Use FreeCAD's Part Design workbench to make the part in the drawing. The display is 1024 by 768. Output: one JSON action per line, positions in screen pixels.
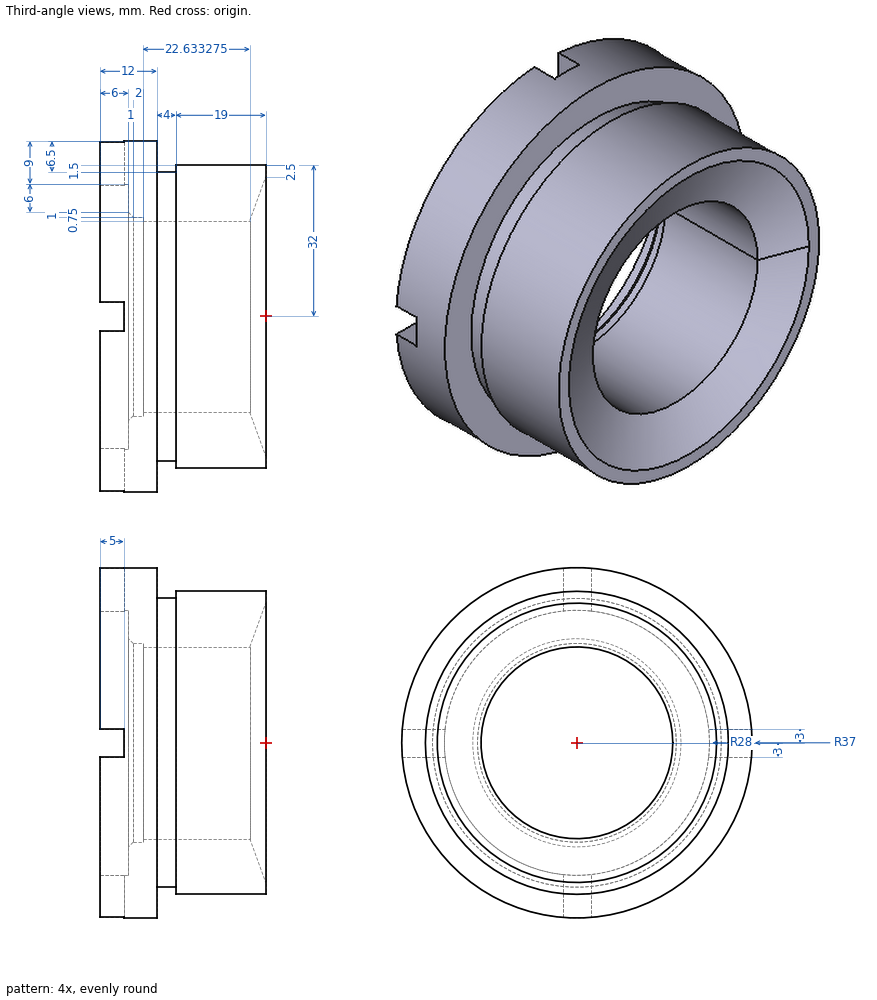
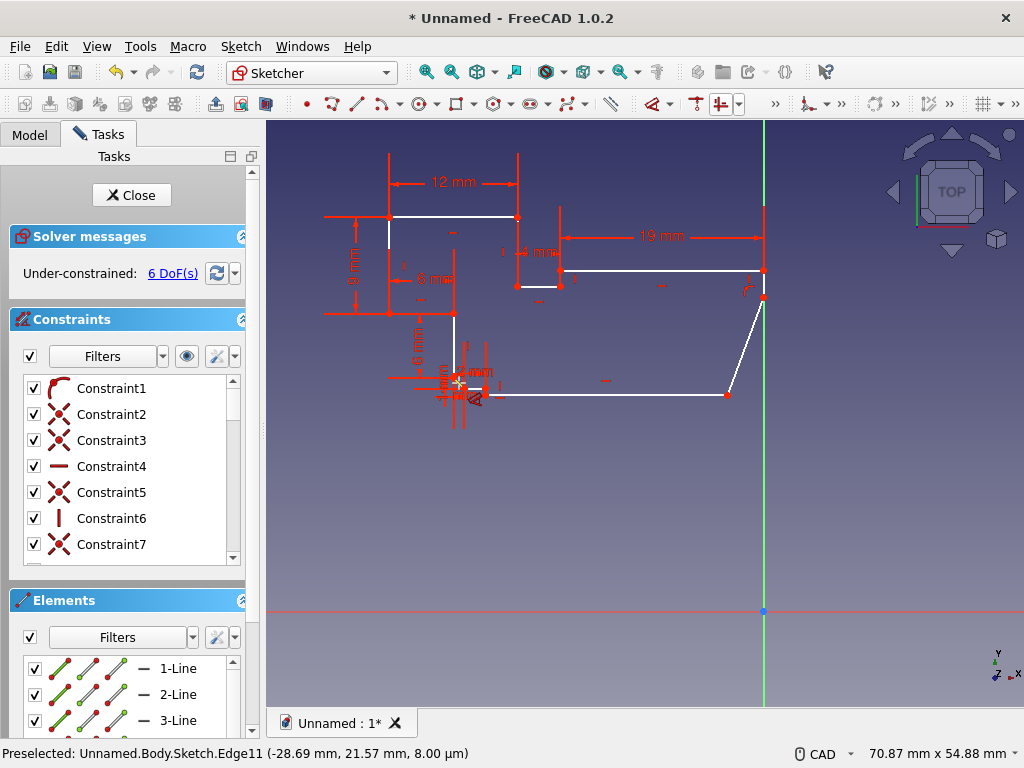
{"action": "scroll", "coordinate": [764, 289], "scroll_direction": "up", "scroll_amount": 3}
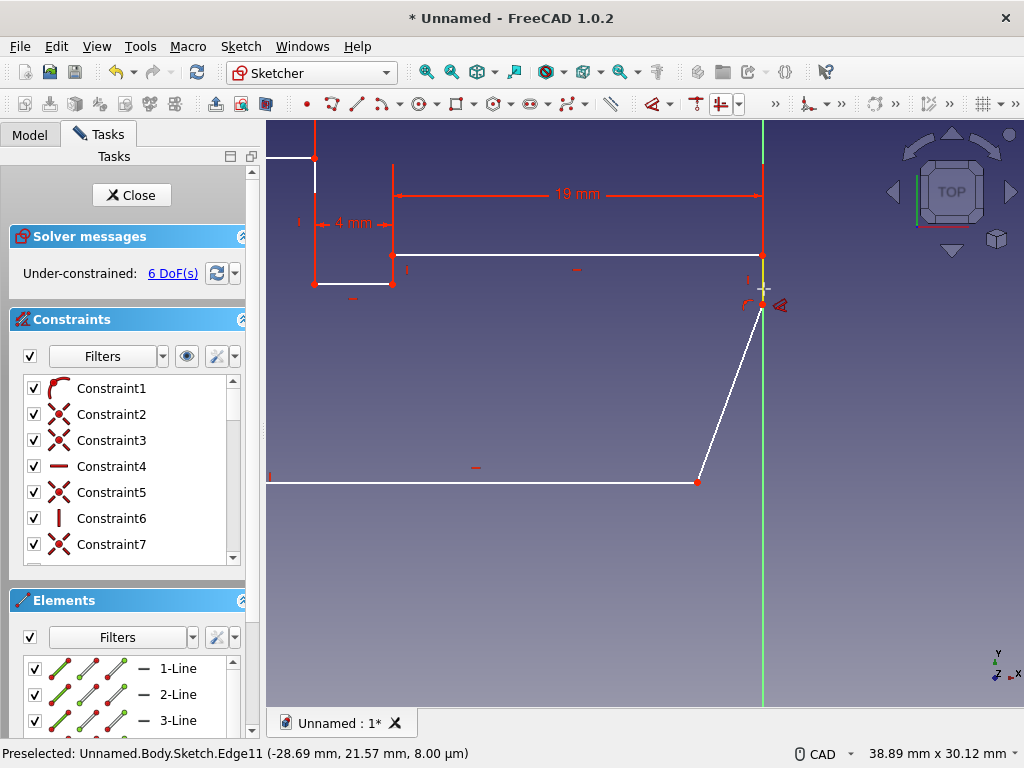
{"action": "left_click", "coordinate": [763, 290]}
{"action": "left_click", "coordinate": [797, 280]}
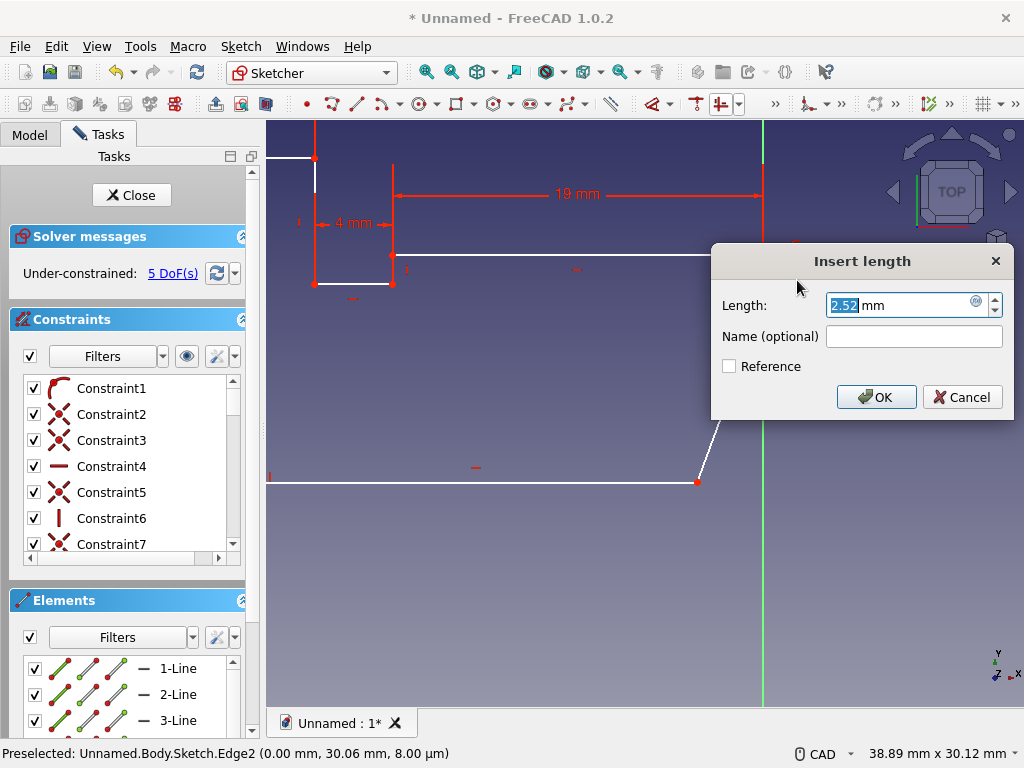
{"action": "type", "text": "2.5"}
{"action": "key", "text": "Return"}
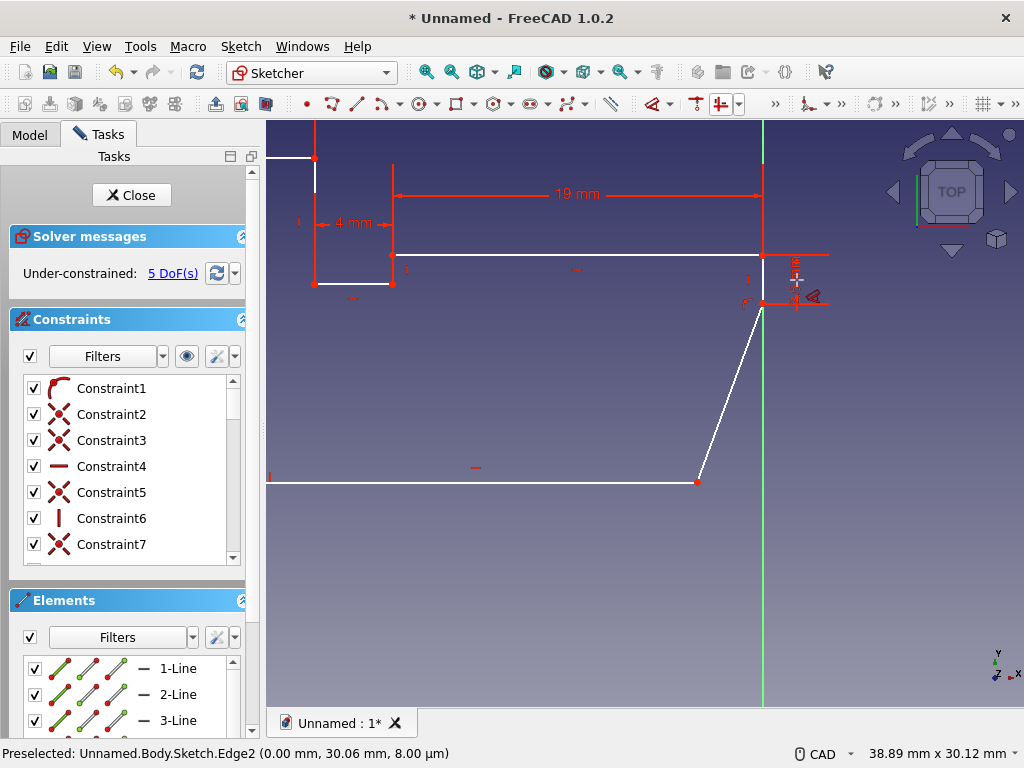
{"action": "scroll", "coordinate": [393, 267], "scroll_direction": "up", "scroll_amount": 2}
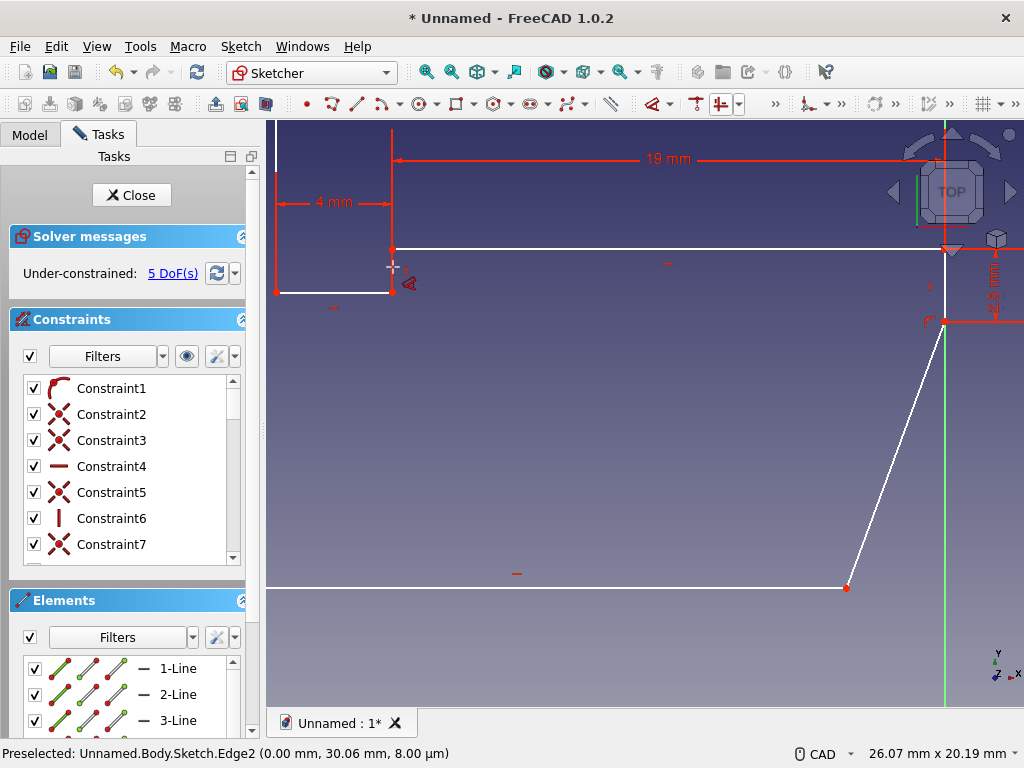
{"action": "left_click", "coordinate": [392, 267]}
{"action": "left_click", "coordinate": [358, 271]}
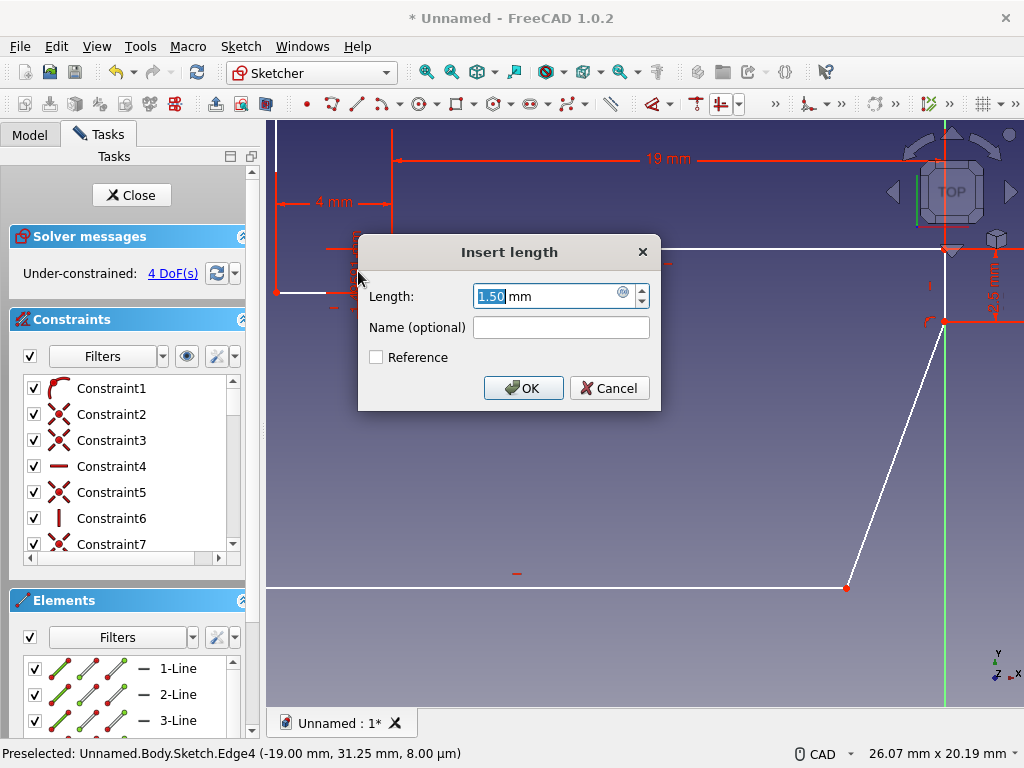
{"action": "type", "text": "1.5"}
{"action": "key", "text": "Return"}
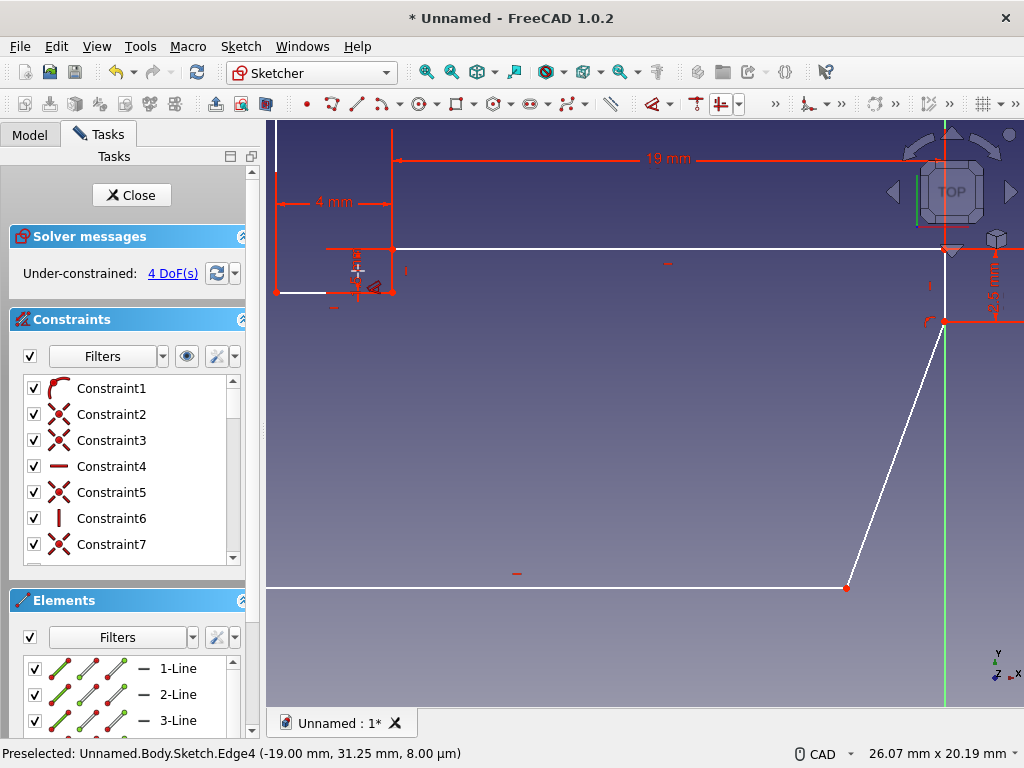
{"action": "scroll", "coordinate": [658, 282], "scroll_direction": "down", "scroll_amount": 5}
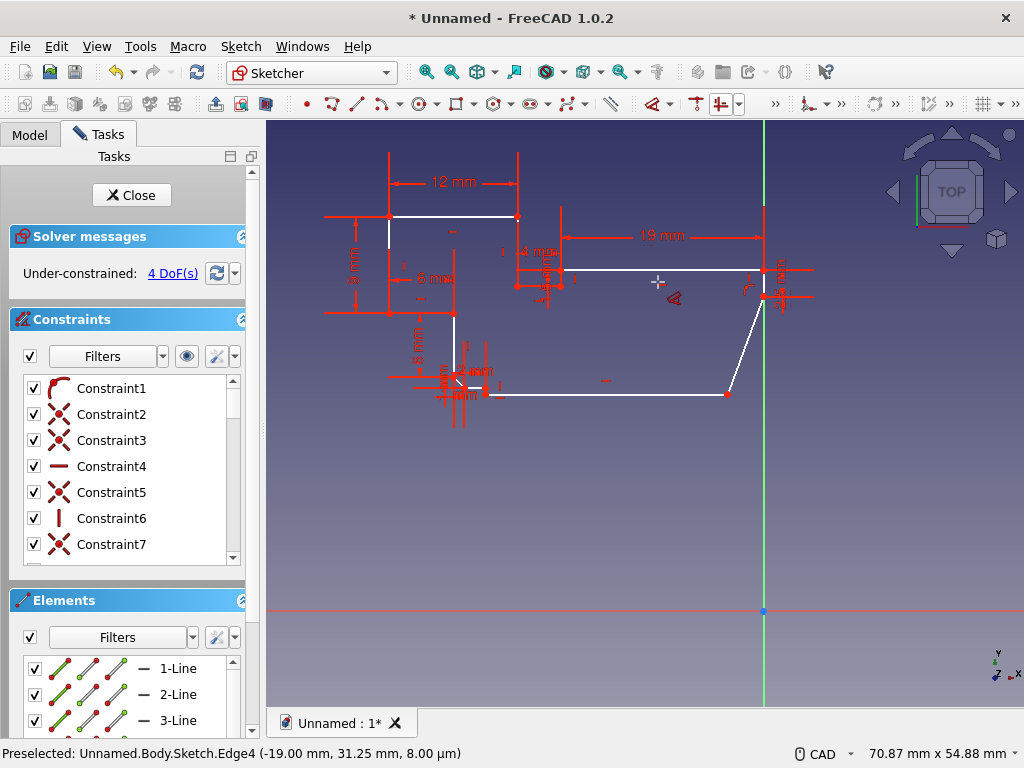
{"action": "left_click", "coordinate": [518, 265]}
{"action": "left_click", "coordinate": [552, 227]}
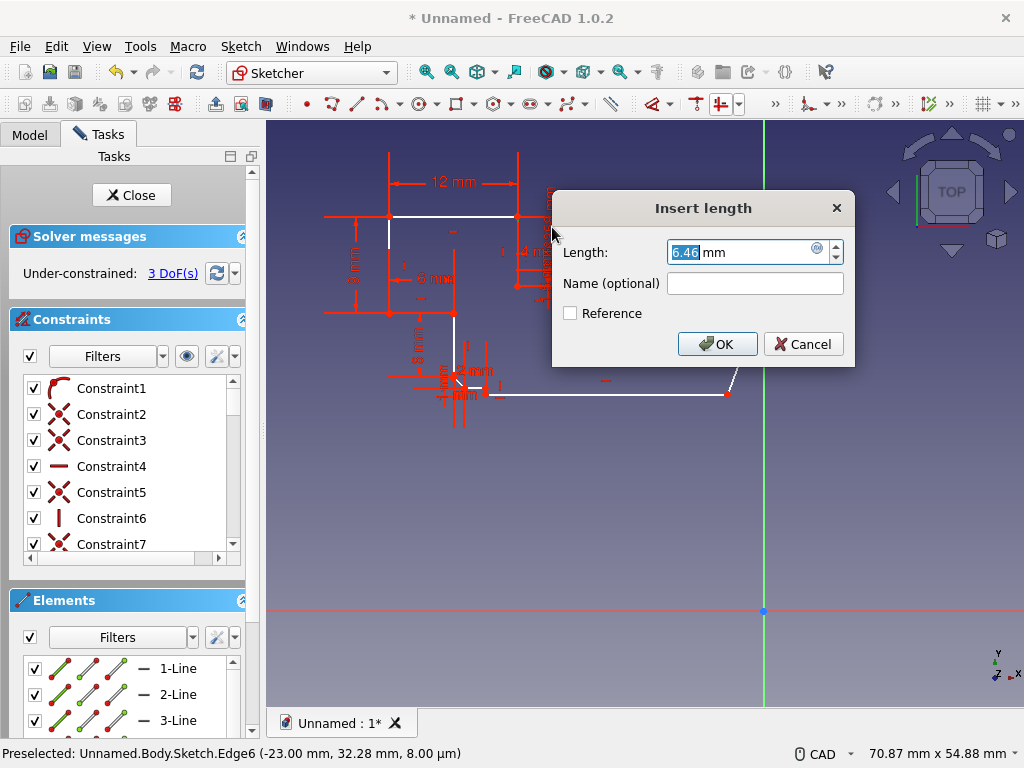
{"action": "type", "text": "6.5"}
{"action": "key", "text": "Return"}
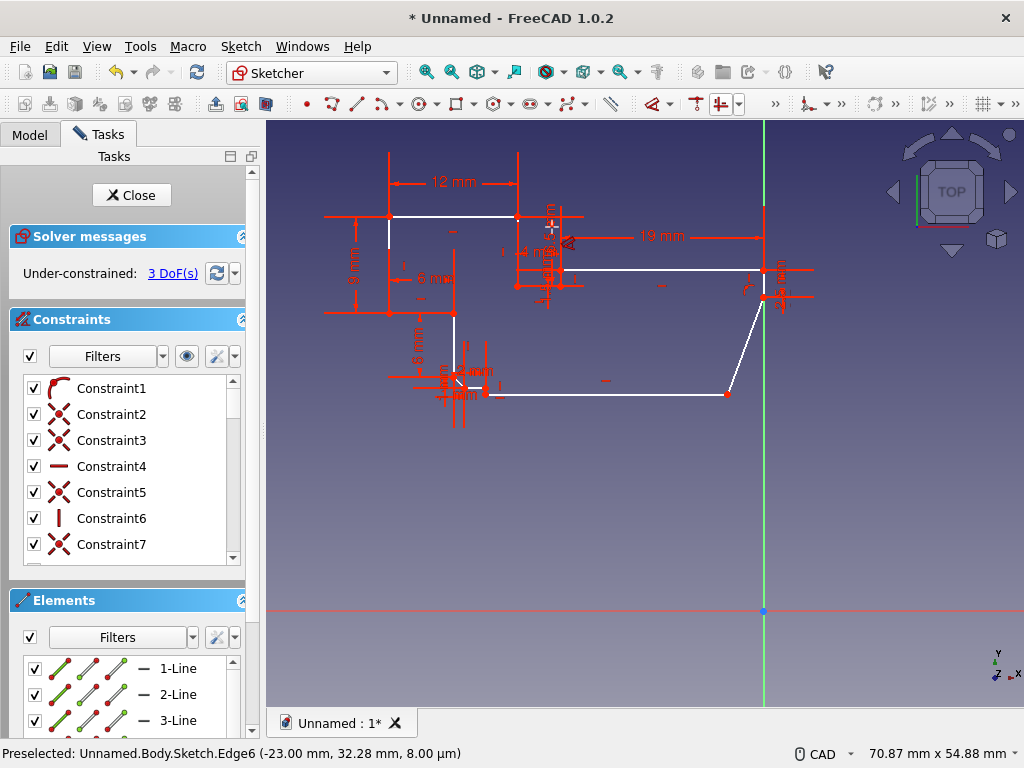
{"action": "left_click", "coordinate": [764, 270]}
{"action": "left_click", "coordinate": [798, 441]}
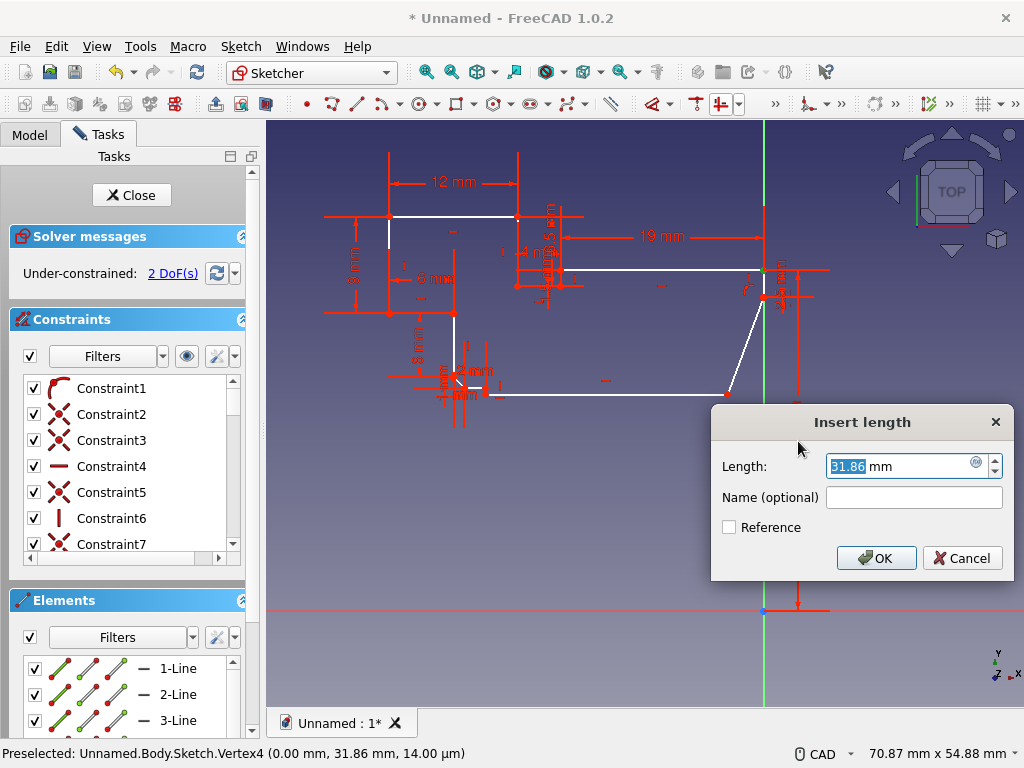
{"action": "type", "text": "32"}
{"action": "key", "text": "Return"}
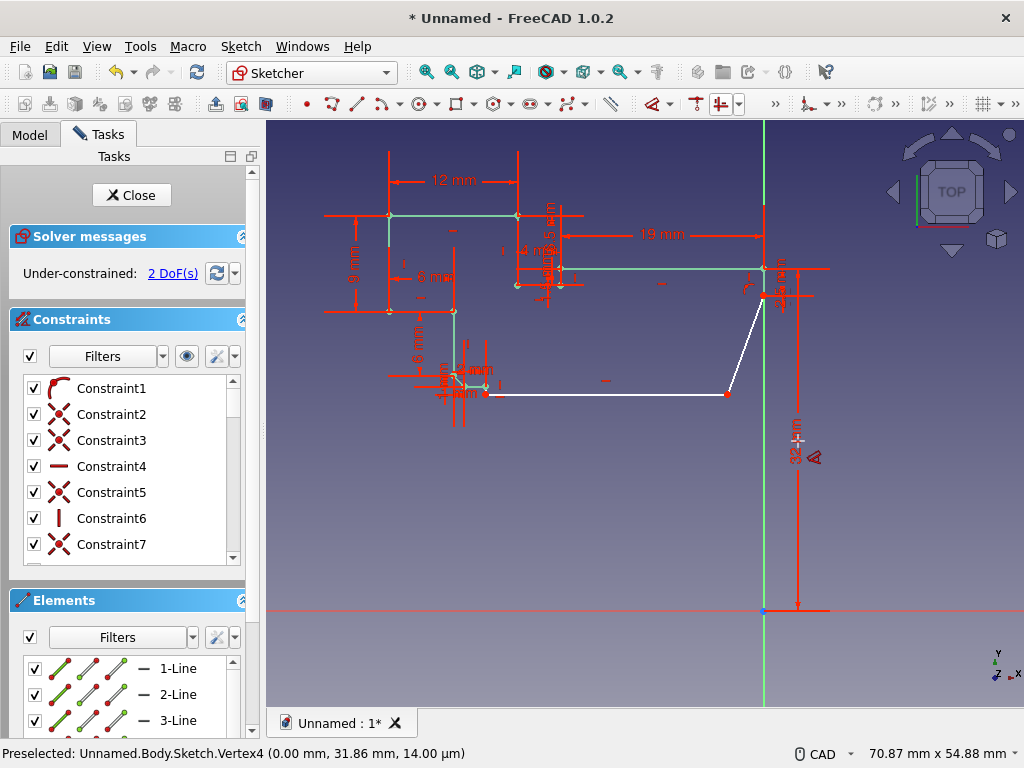
{"action": "scroll", "coordinate": [486, 391], "scroll_direction": "up", "scroll_amount": 8}